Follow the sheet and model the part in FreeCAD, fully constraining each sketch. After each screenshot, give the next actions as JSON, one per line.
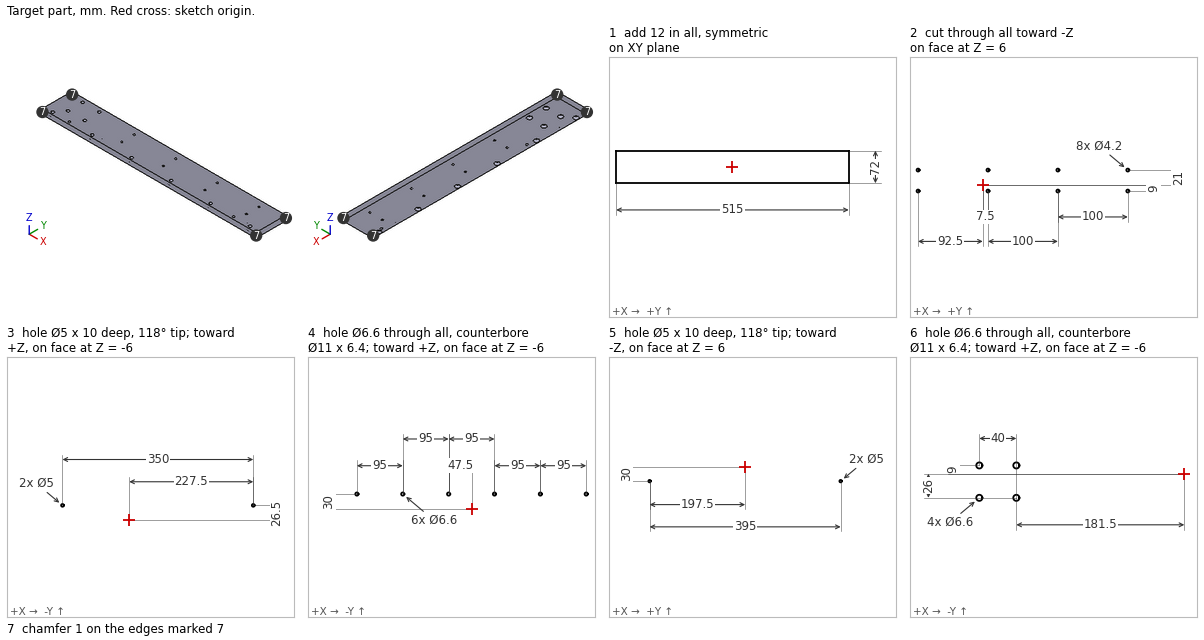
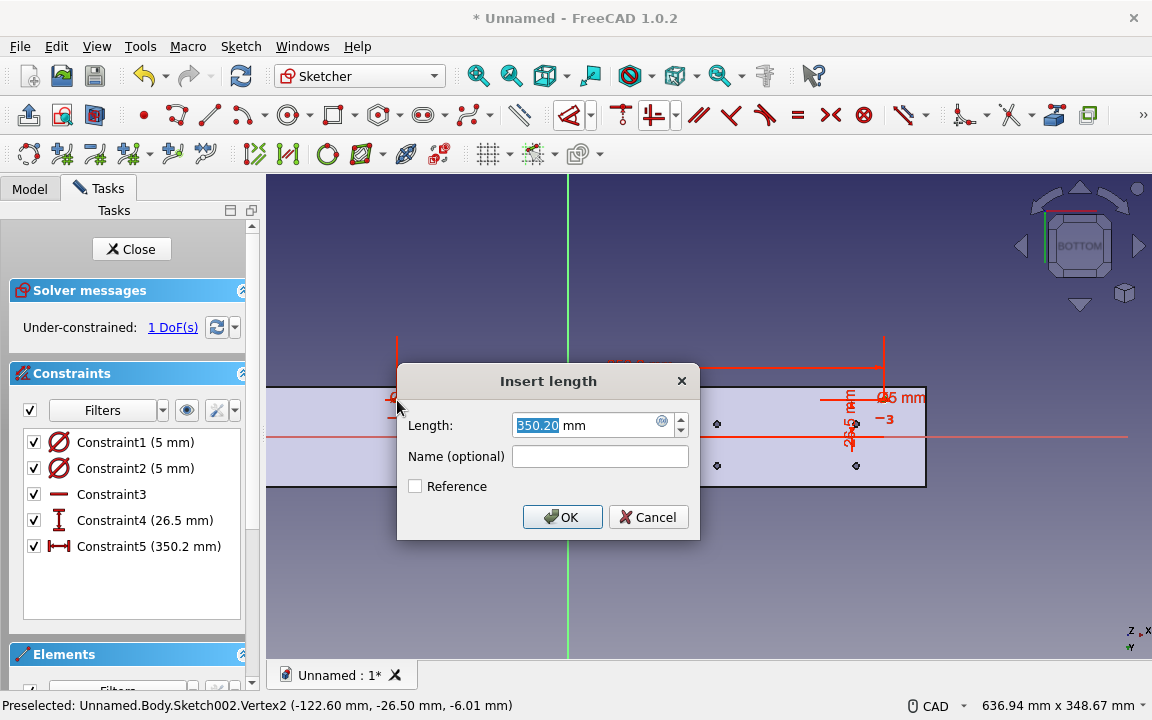
{"action": "type", "text": "350"}
{"action": "key", "text": "Return"}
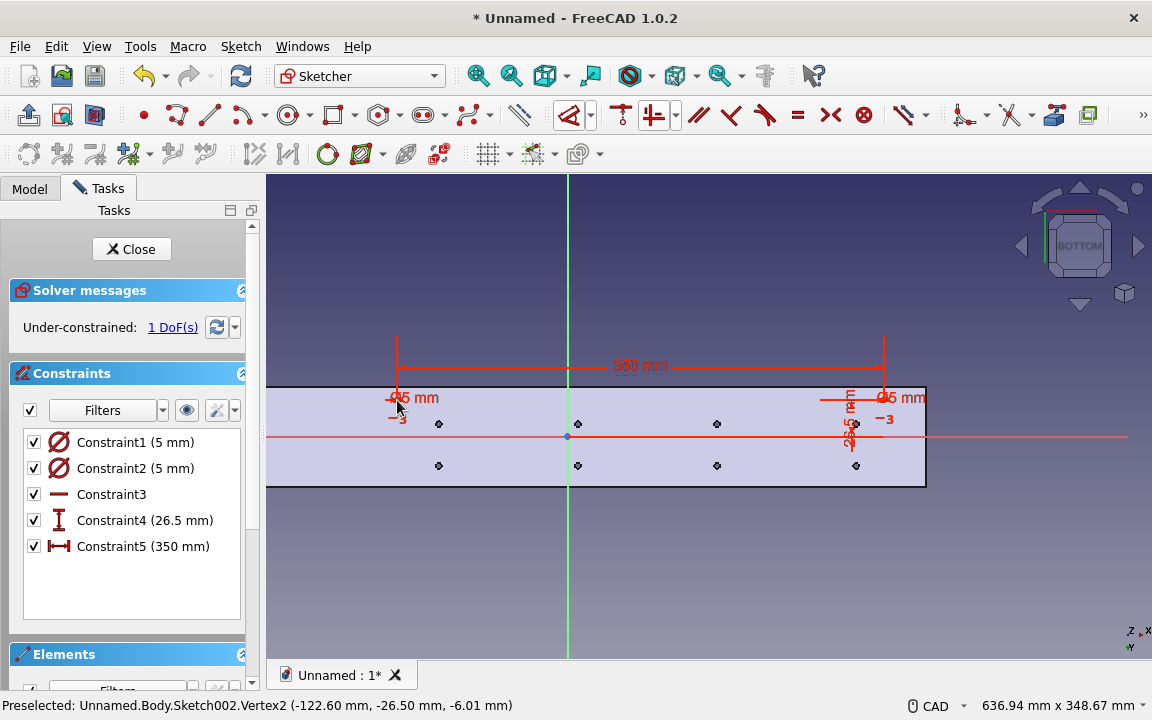
{"action": "left_click", "coordinate": [884, 400]}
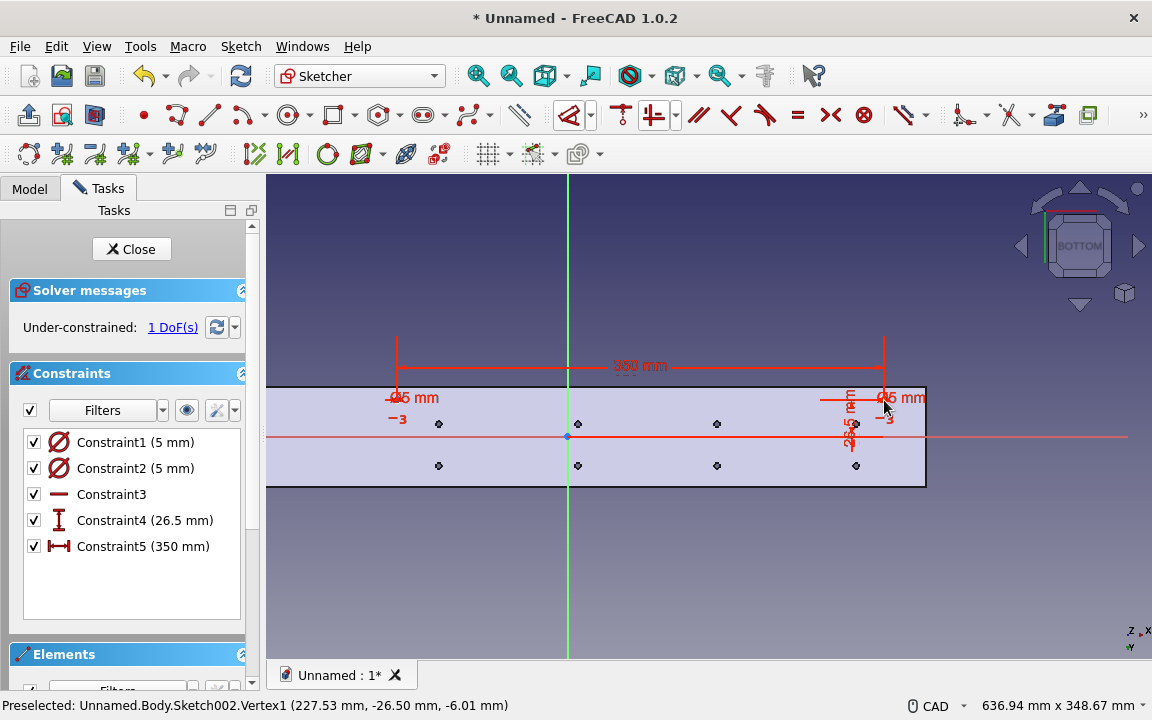
{"action": "left_click", "coordinate": [590, 116]}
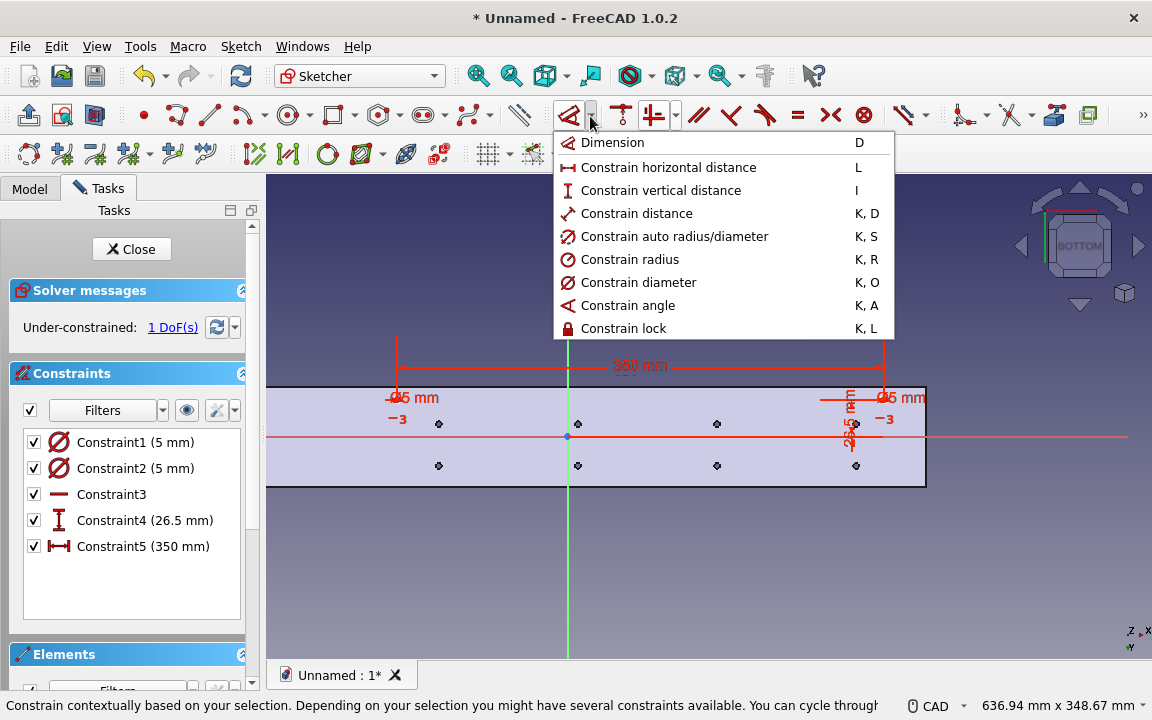
{"action": "left_click", "coordinate": [724, 168]}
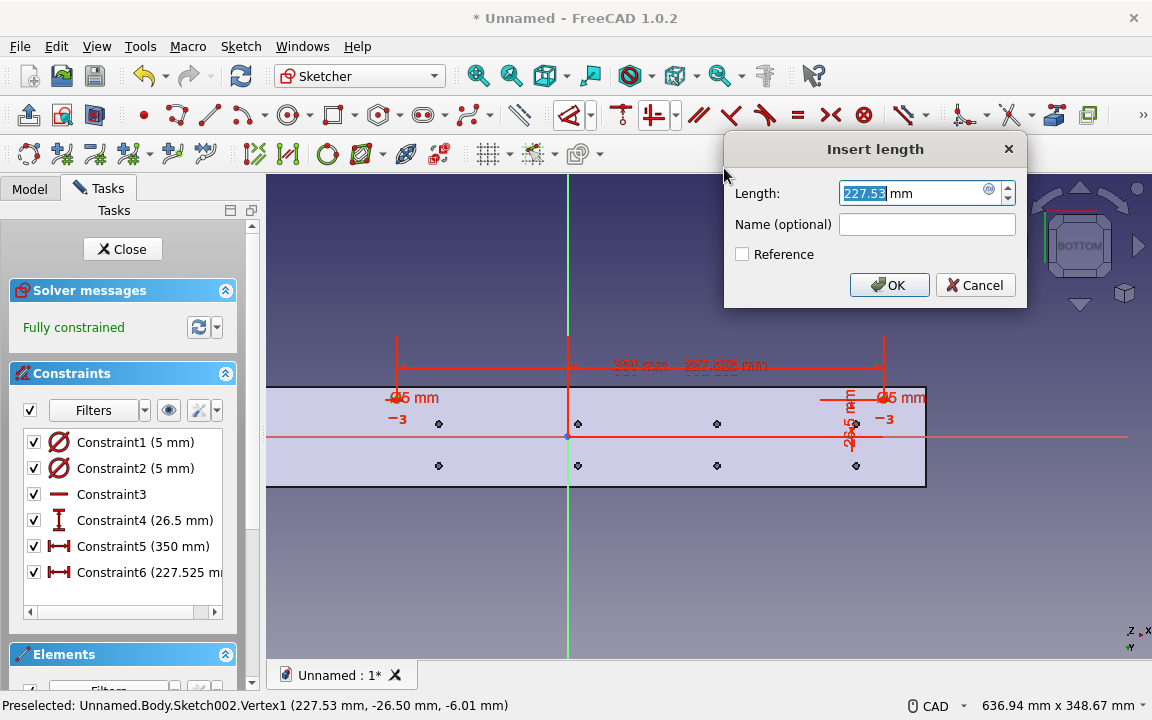
{"action": "type", "text": "227.5"}
{"action": "key", "text": "Return"}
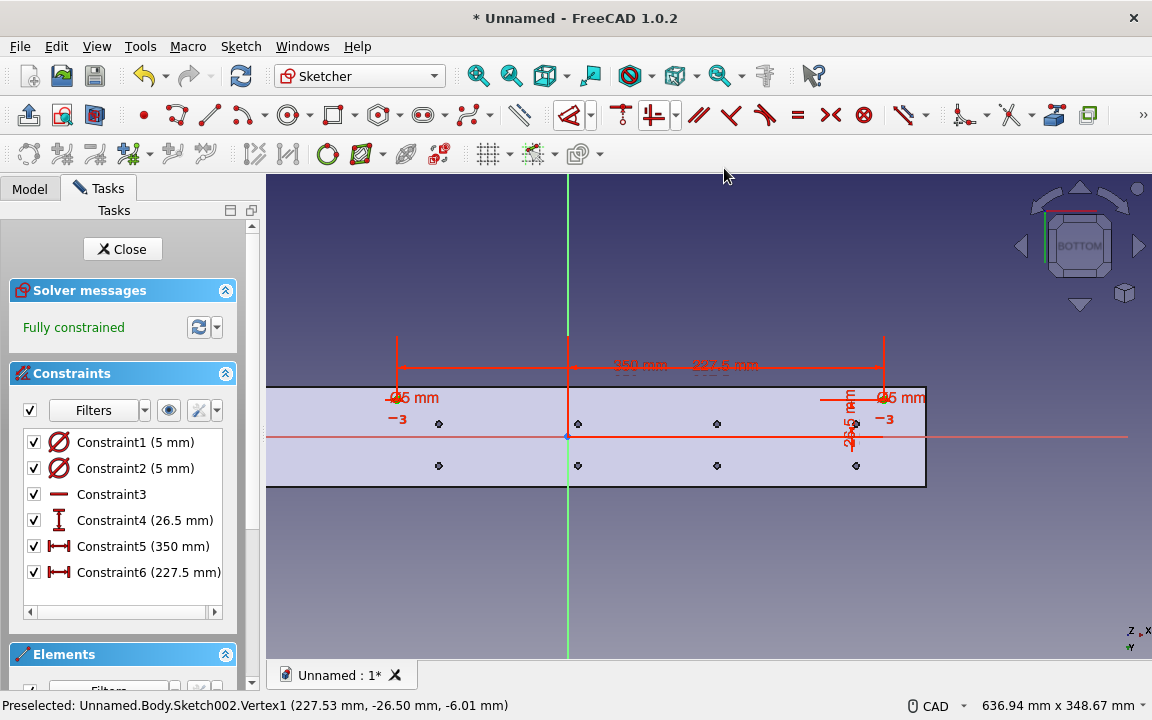
{"action": "left_click", "coordinate": [123, 249]}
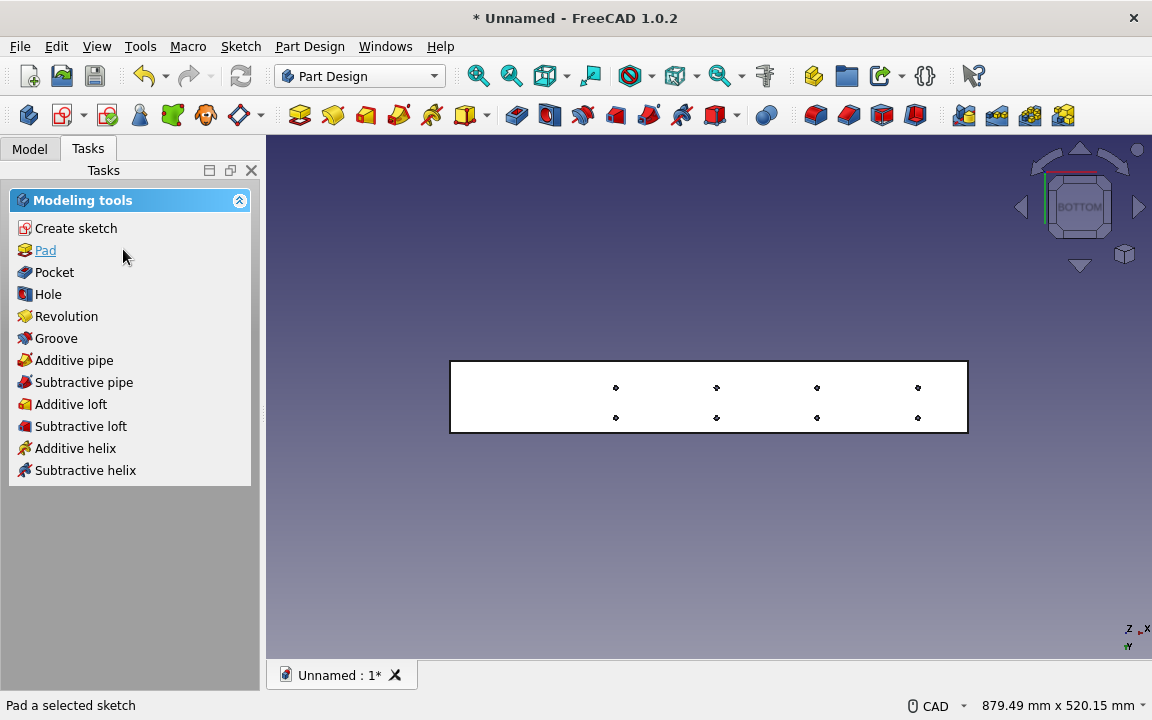
{"action": "left_click", "coordinate": [550, 116]}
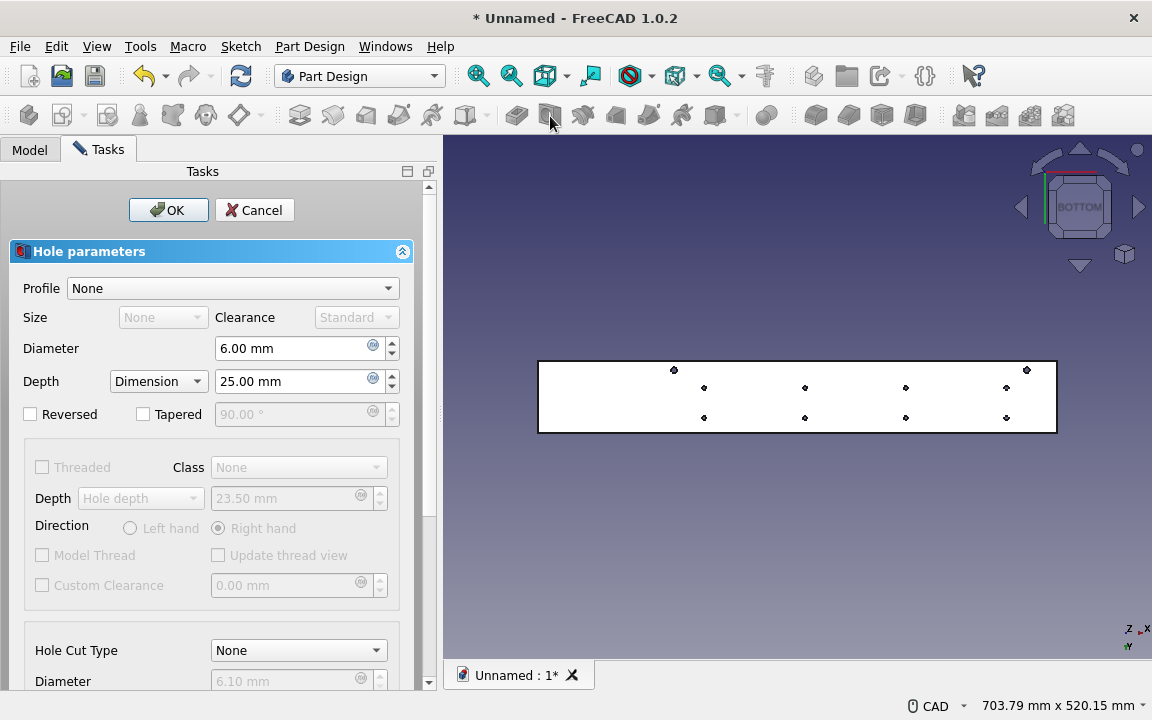
{"action": "triple_click", "coordinate": [300, 348]}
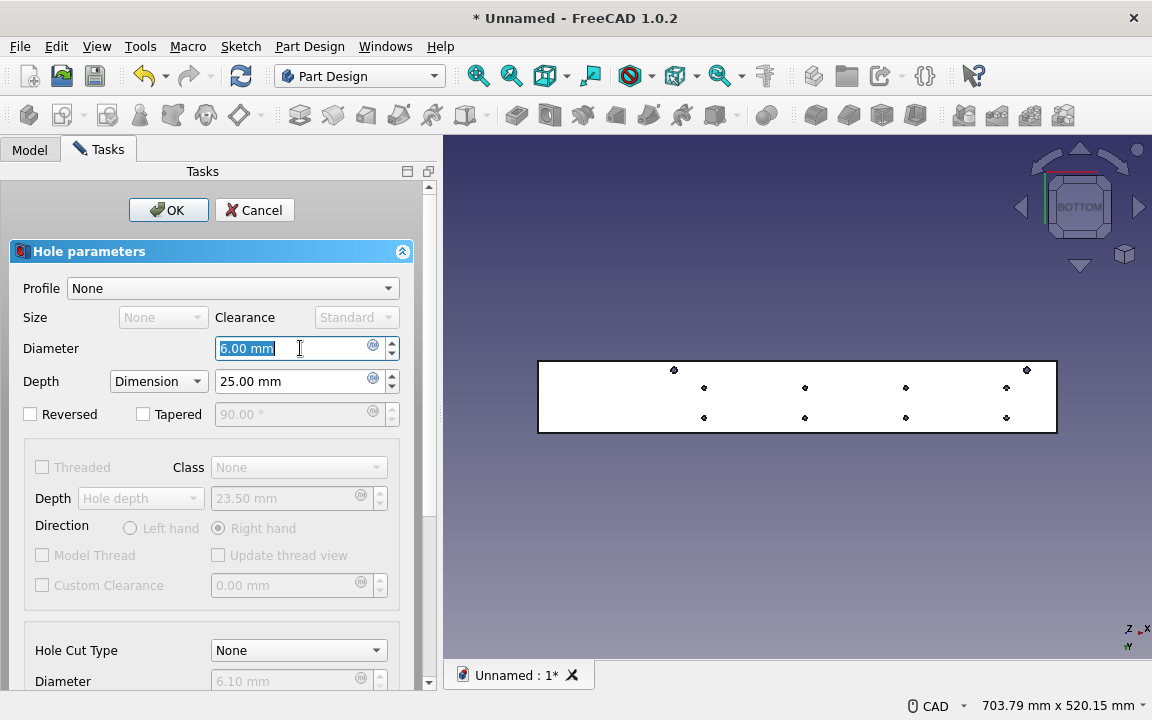
{"action": "type", "text": "5"}
{"action": "key", "text": "Tab"}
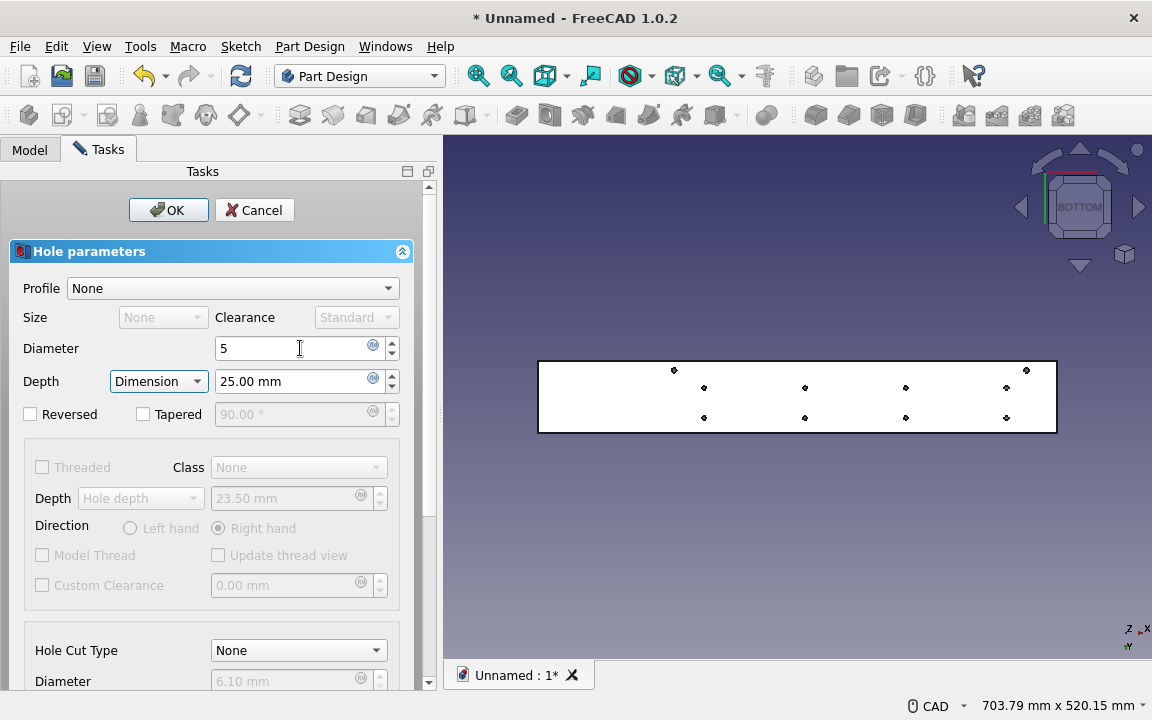
{"action": "triple_click", "coordinate": [300, 382]}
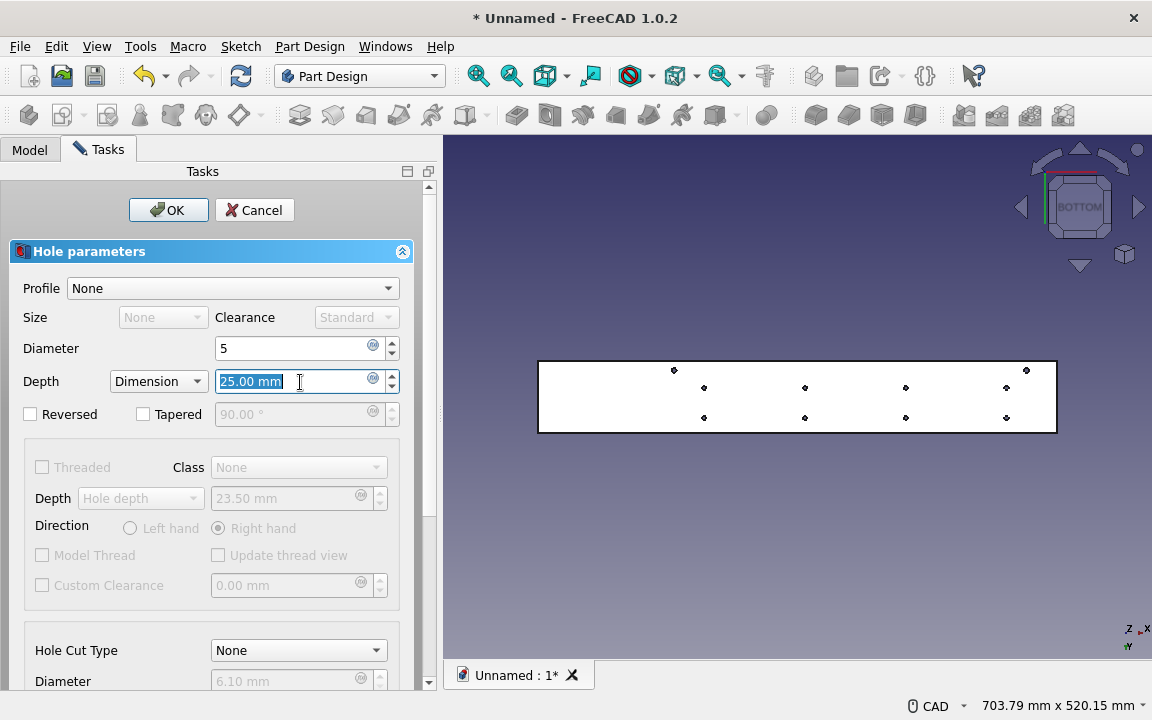
{"action": "type", "text": "10"}
{"action": "key", "text": "Tab"}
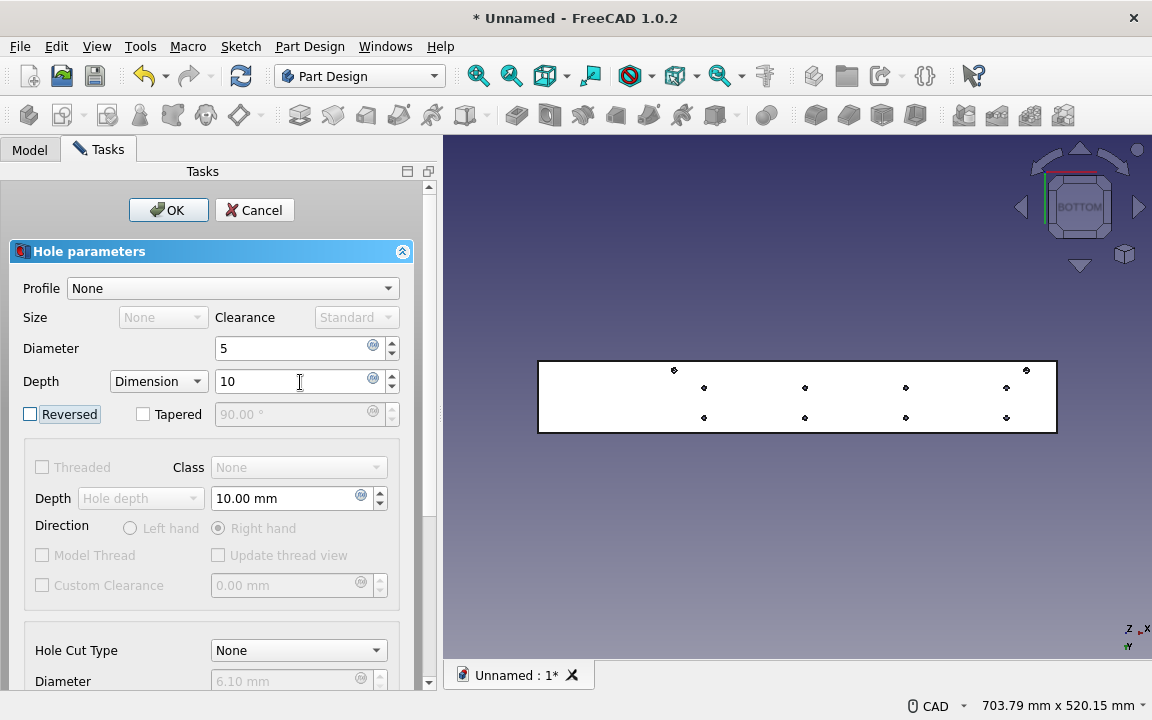
{"action": "left_click", "coordinate": [169, 210]}